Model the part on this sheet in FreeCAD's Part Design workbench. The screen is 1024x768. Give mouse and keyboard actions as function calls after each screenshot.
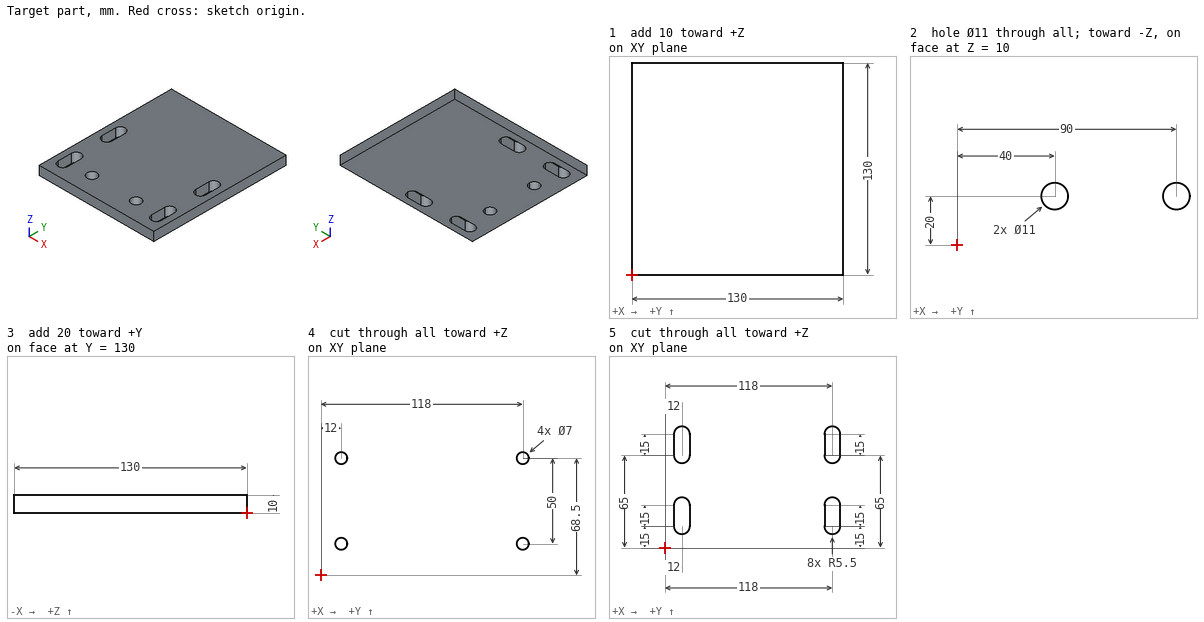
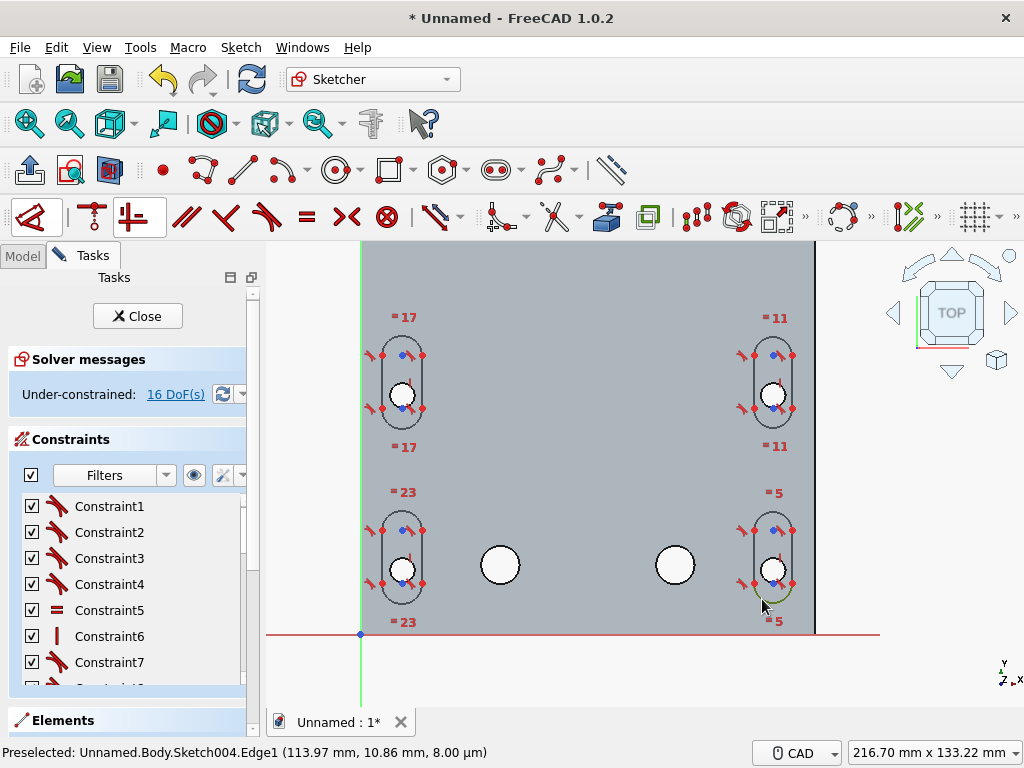
click(762, 424)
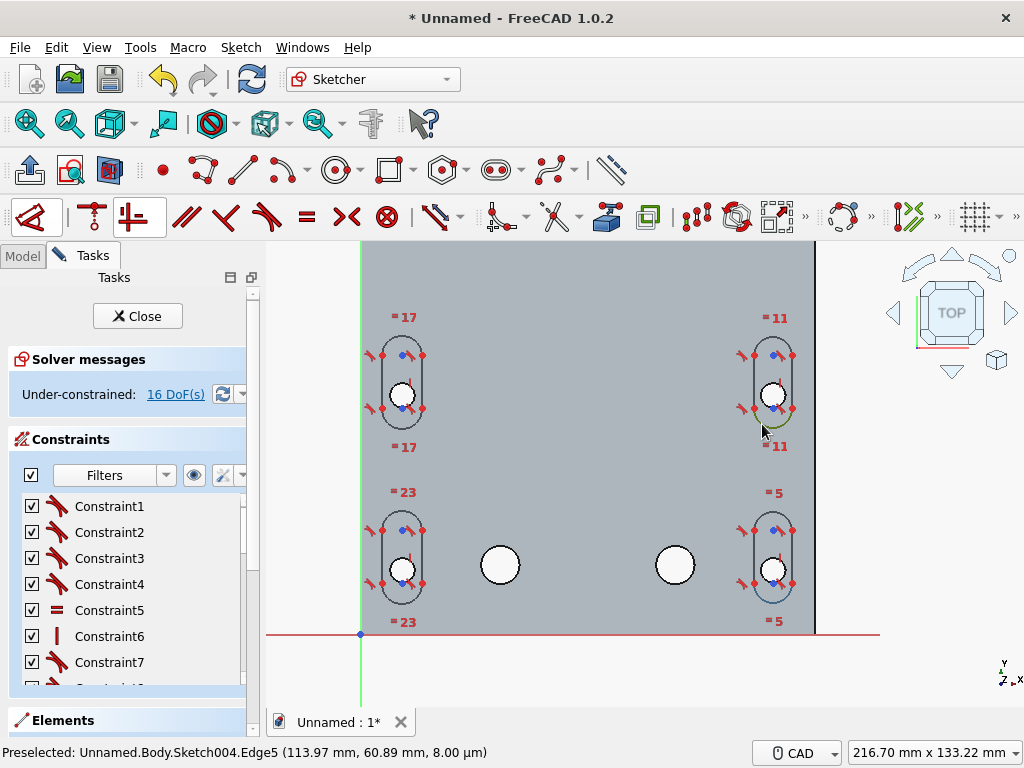
click(390, 425)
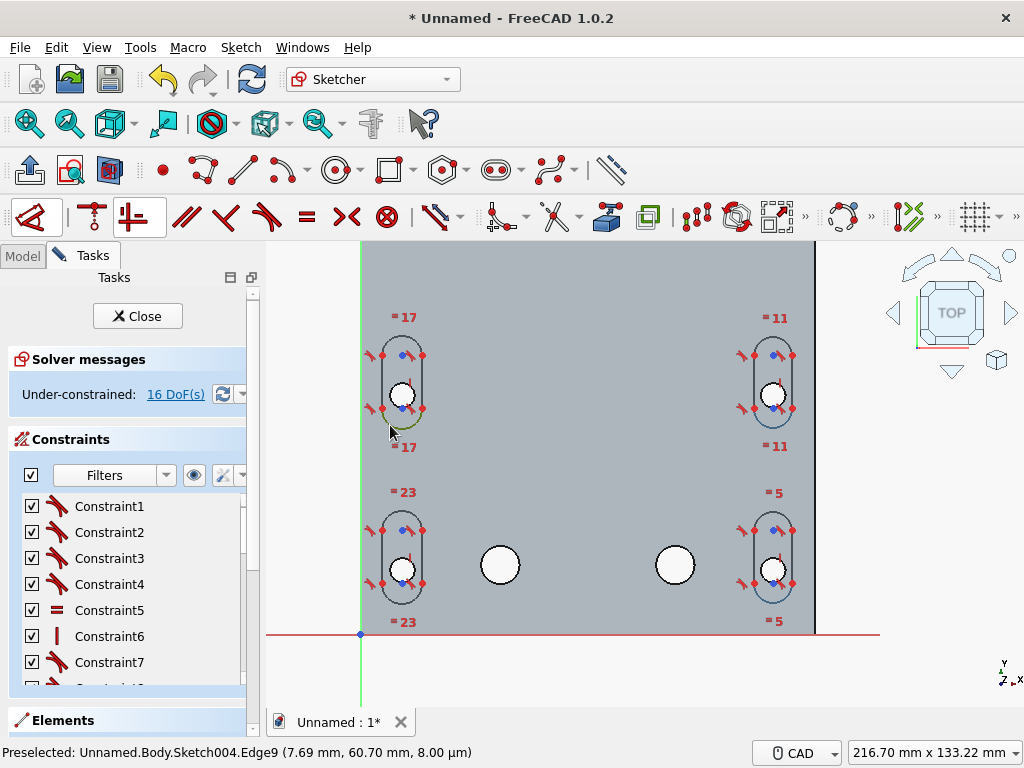
click(390, 600)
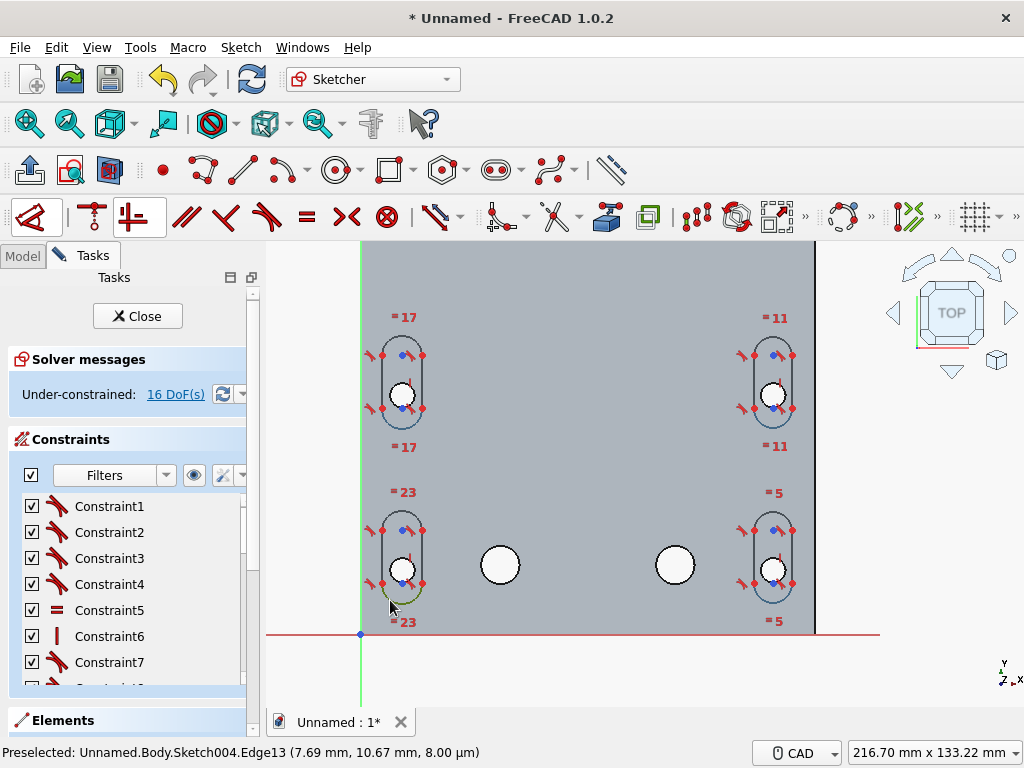
click(308, 218)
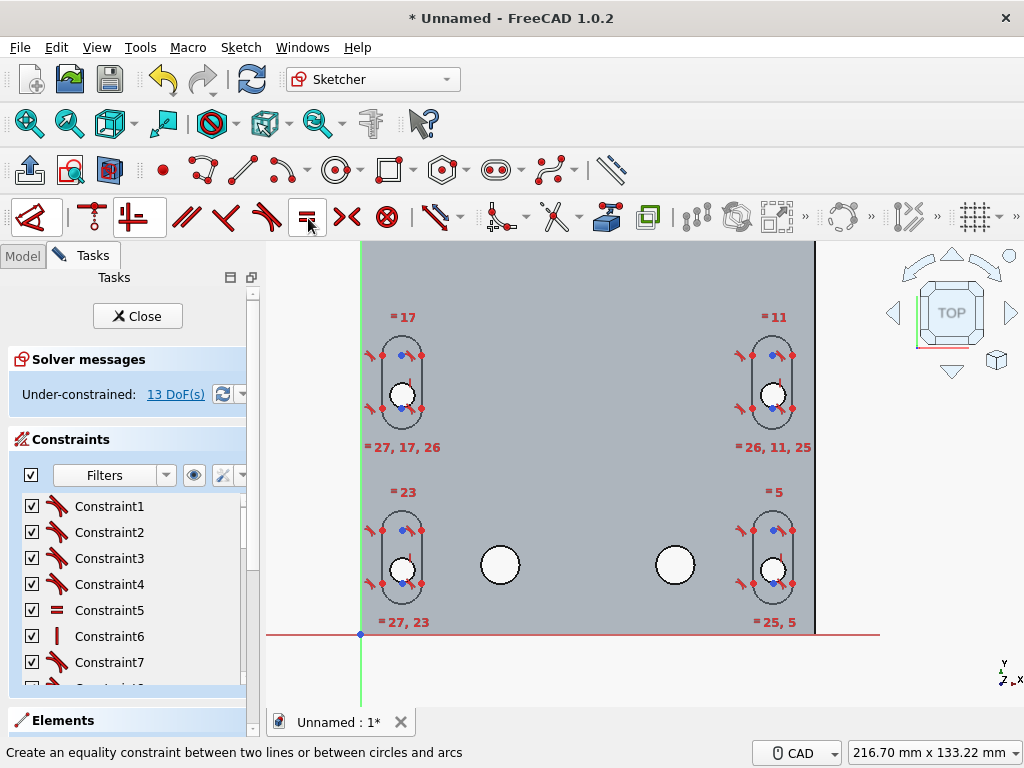
scroll(761, 600, up, 4)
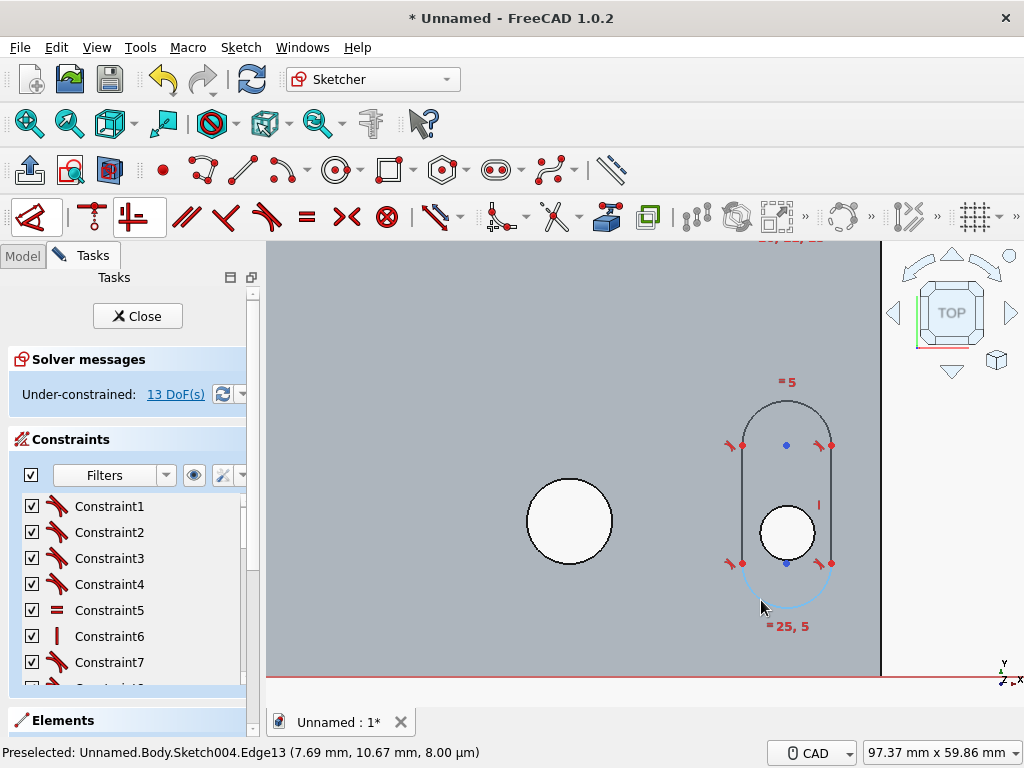
click(761, 599)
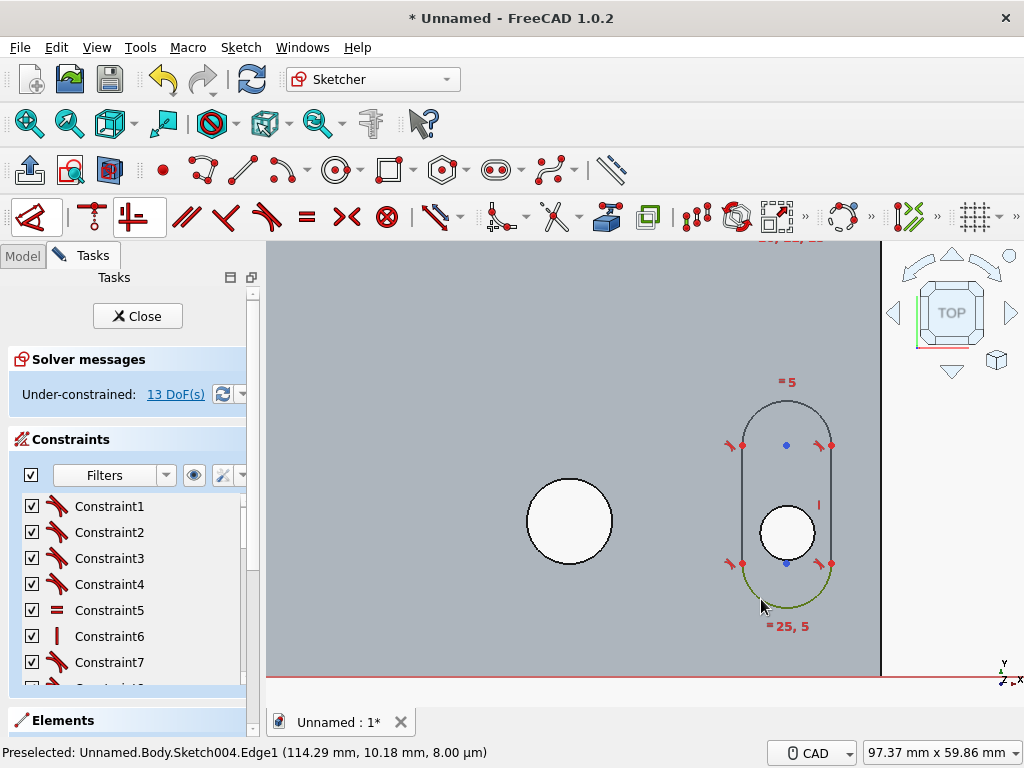
key(k)
key(r)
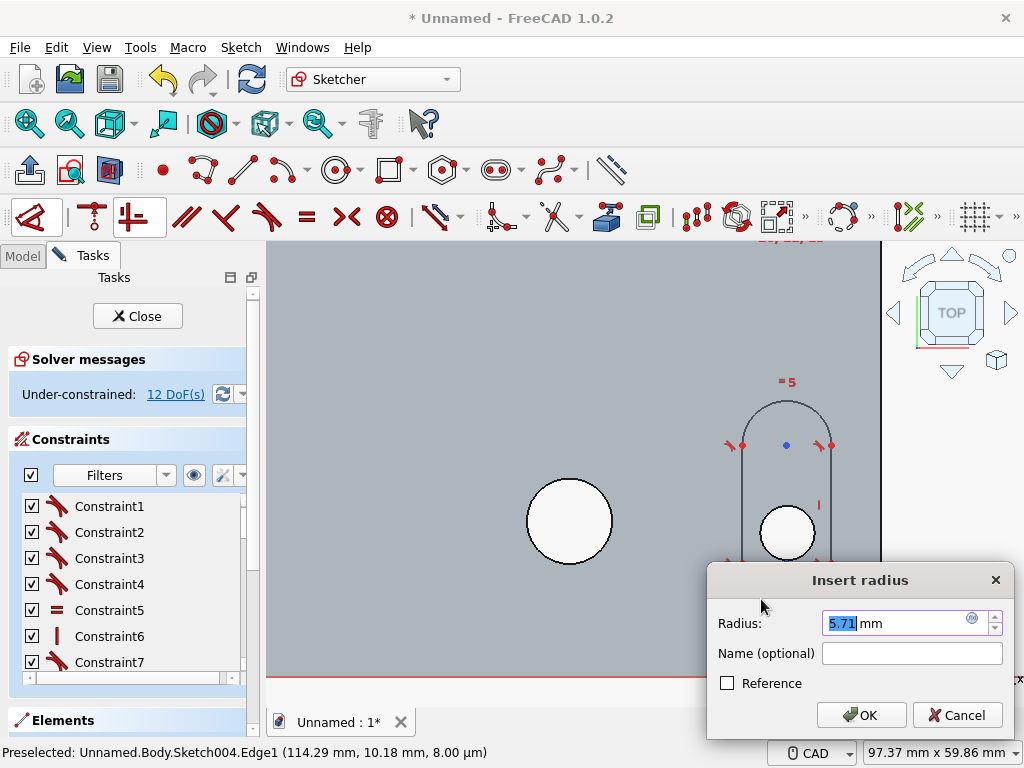
text(5.5)
key(Return)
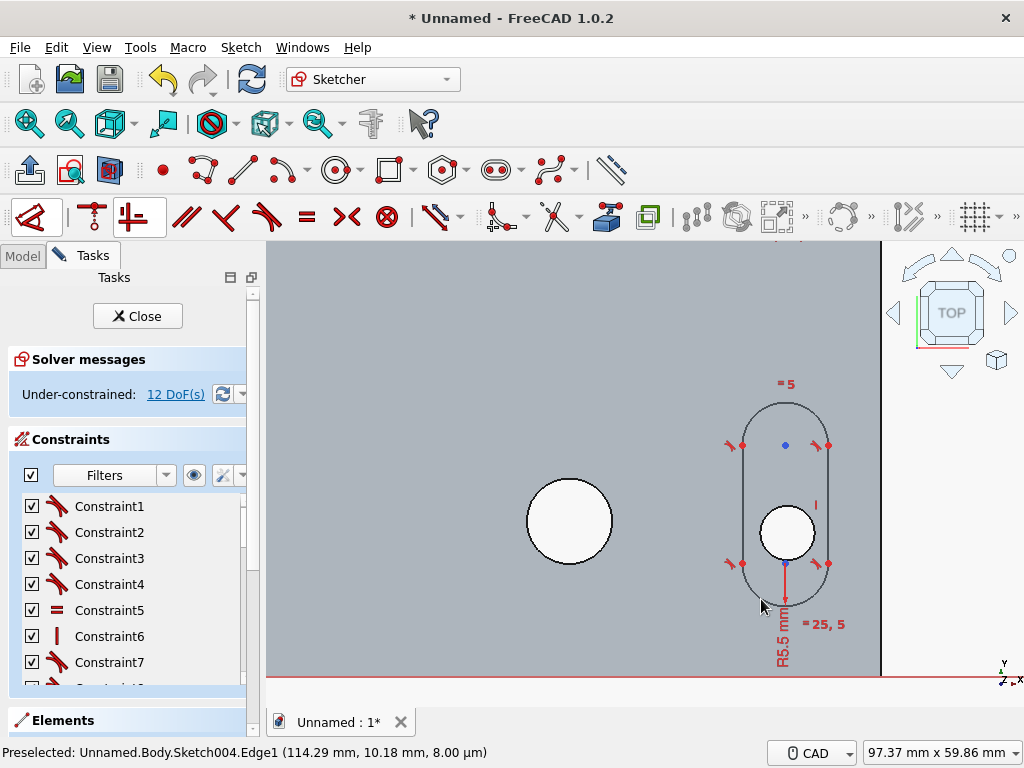
click(743, 528)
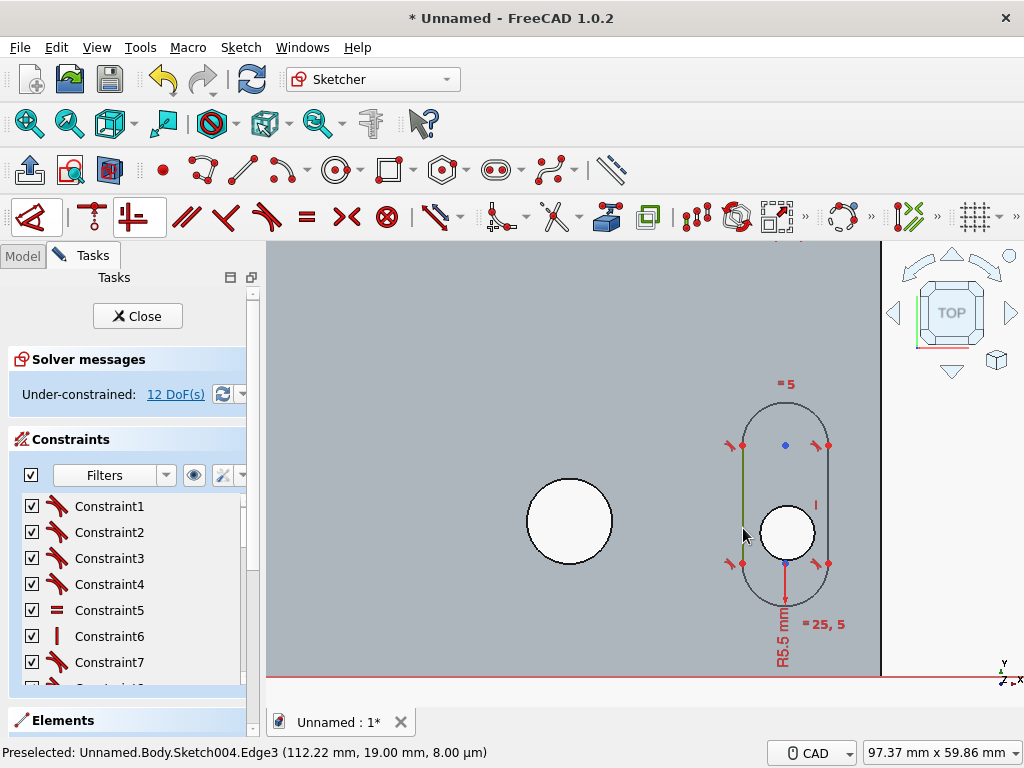
key(i)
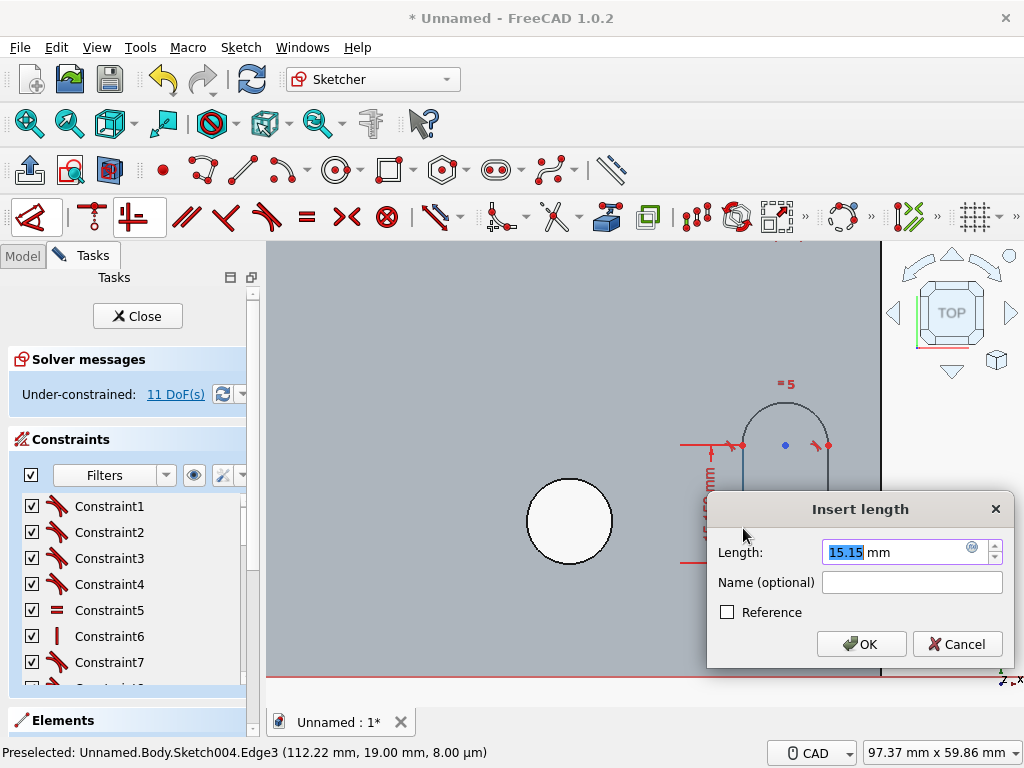
text(15)
key(Return)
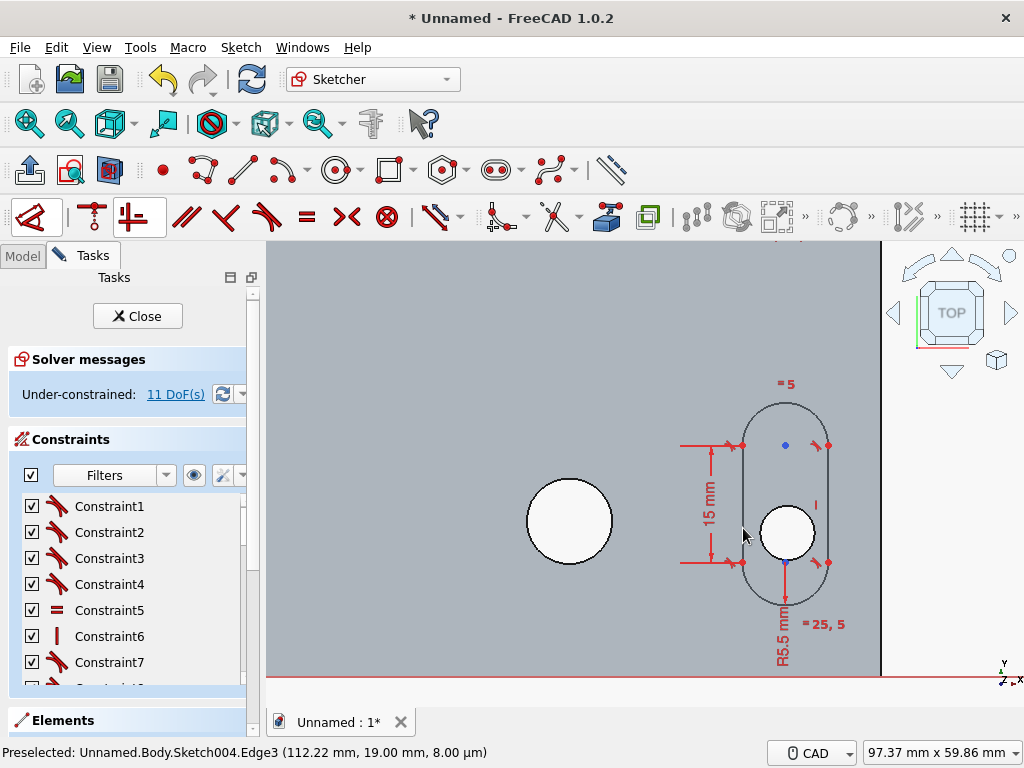
scroll(762, 580, down, 4)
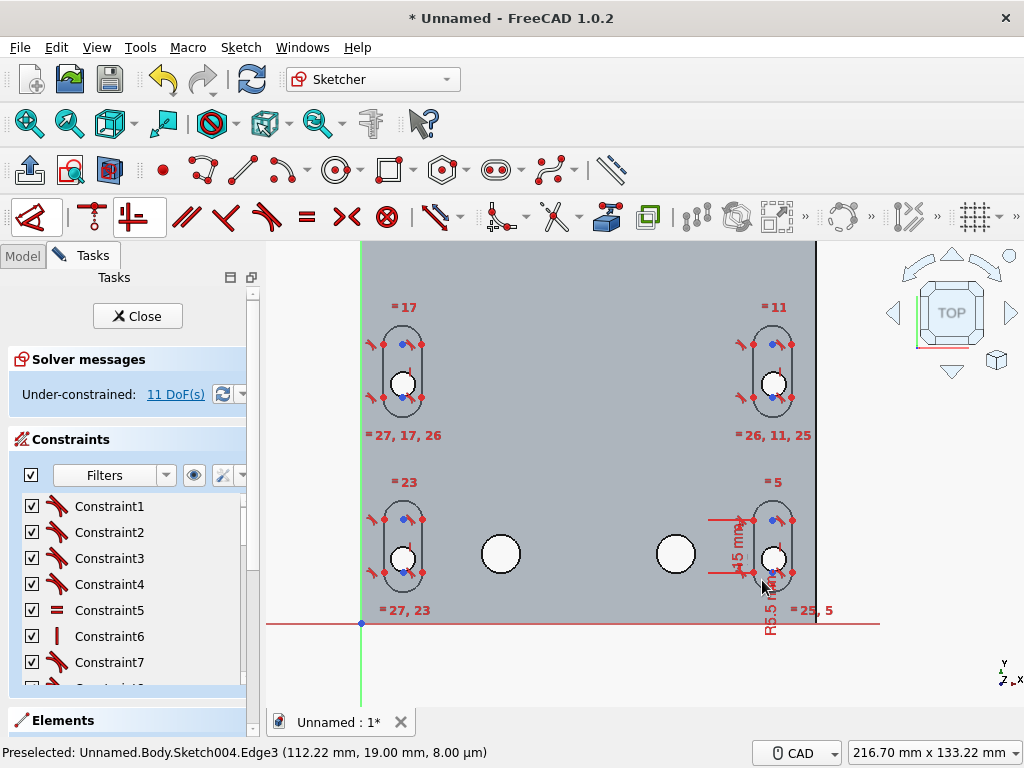
click(754, 382)